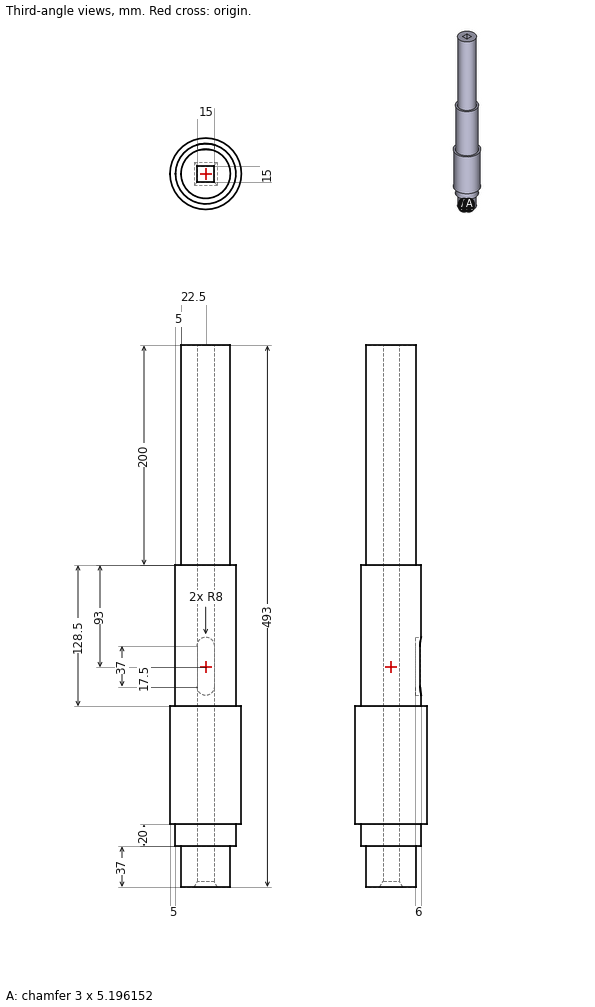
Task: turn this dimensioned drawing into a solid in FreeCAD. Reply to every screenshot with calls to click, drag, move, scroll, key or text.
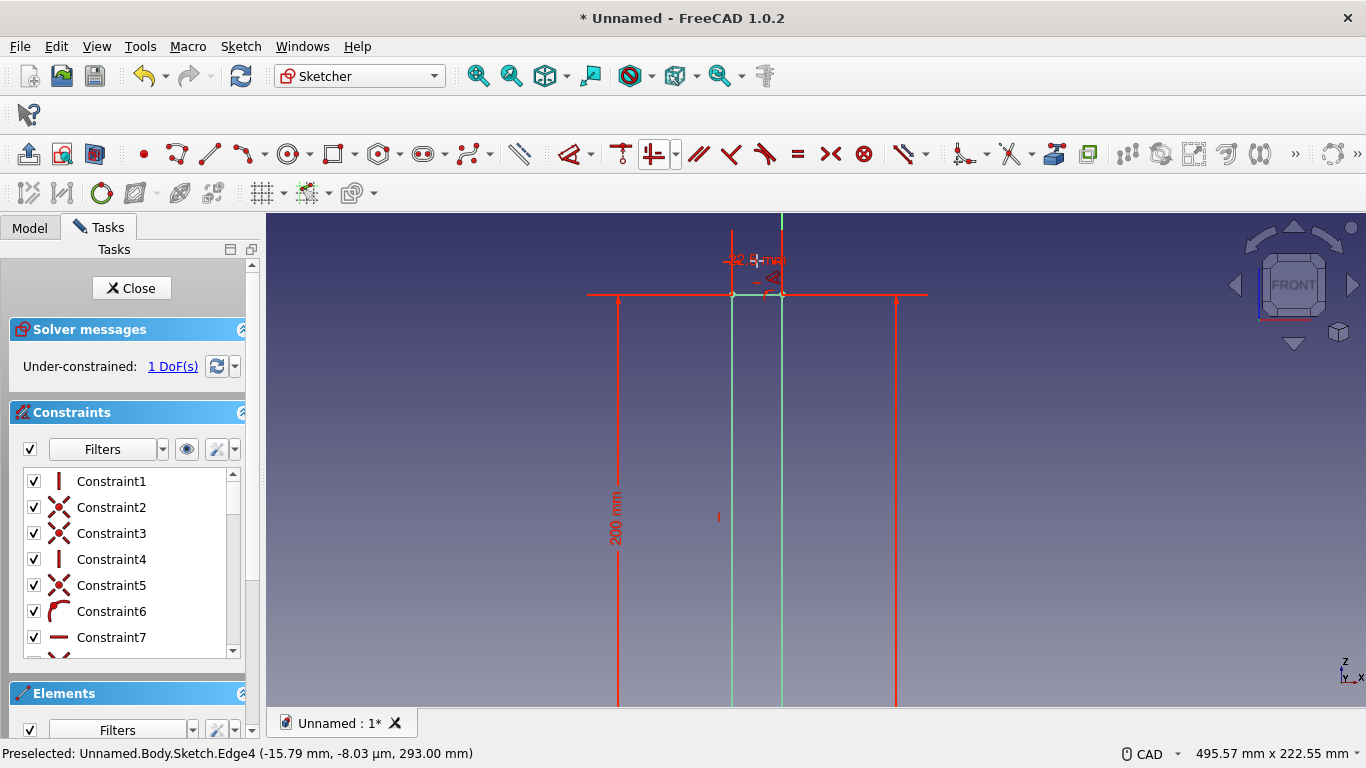
scroll(748, 295, down, 6)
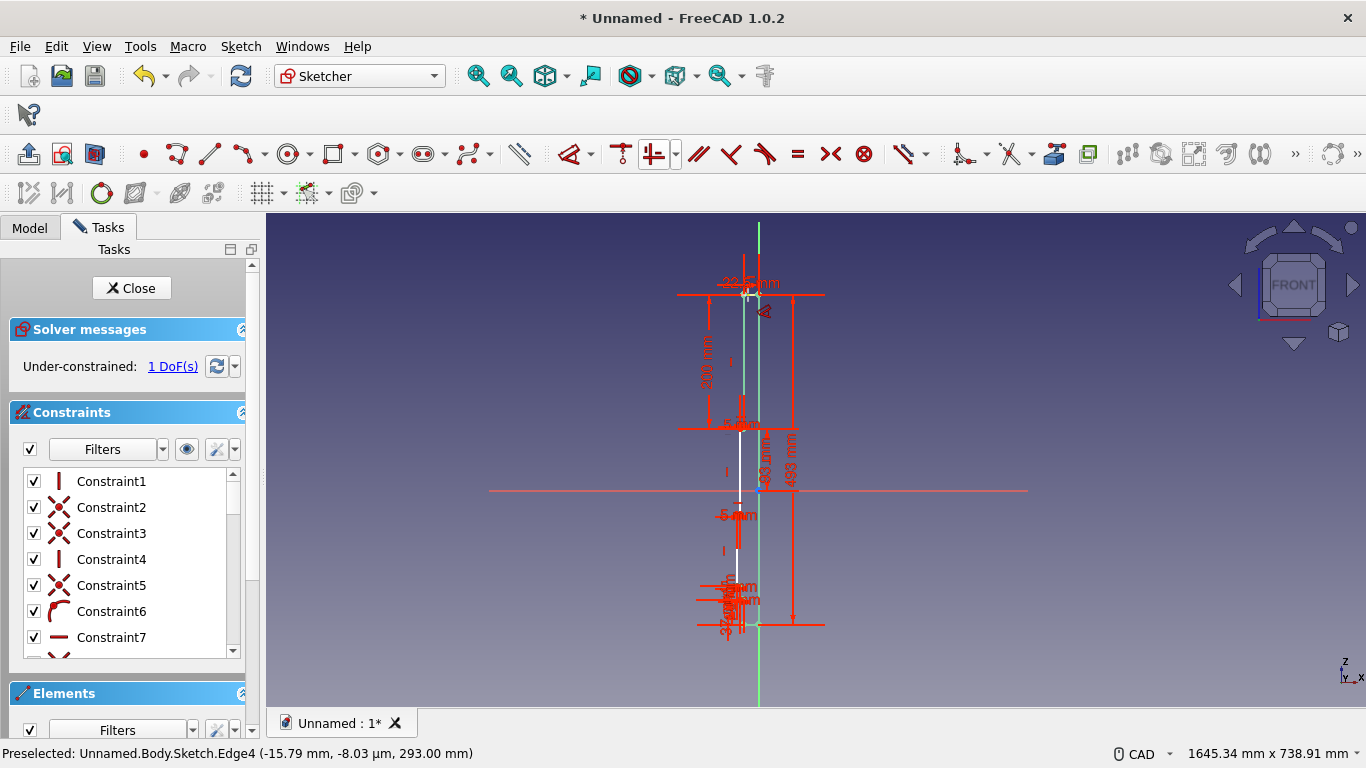
click(740, 454)
click(682, 472)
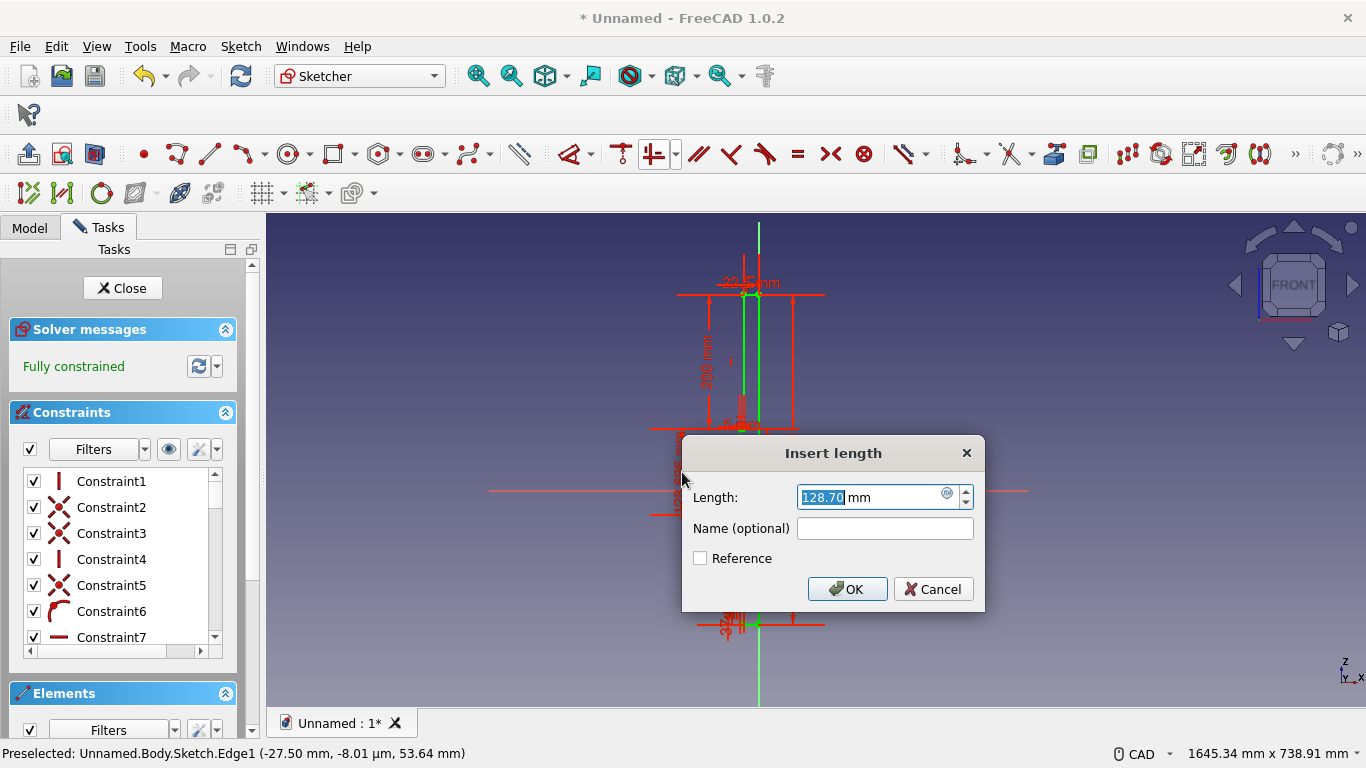
text(128.5)
key(Return)
key(Escape)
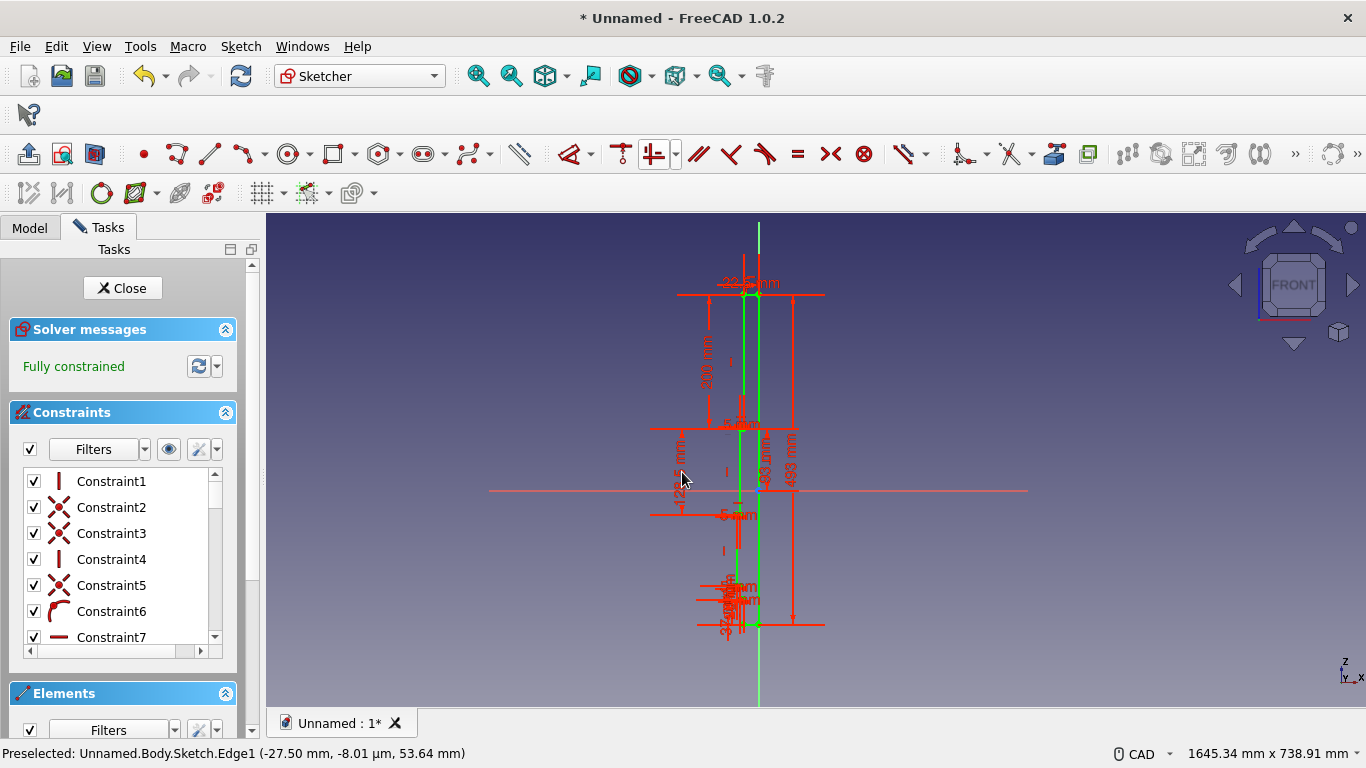
click(123, 288)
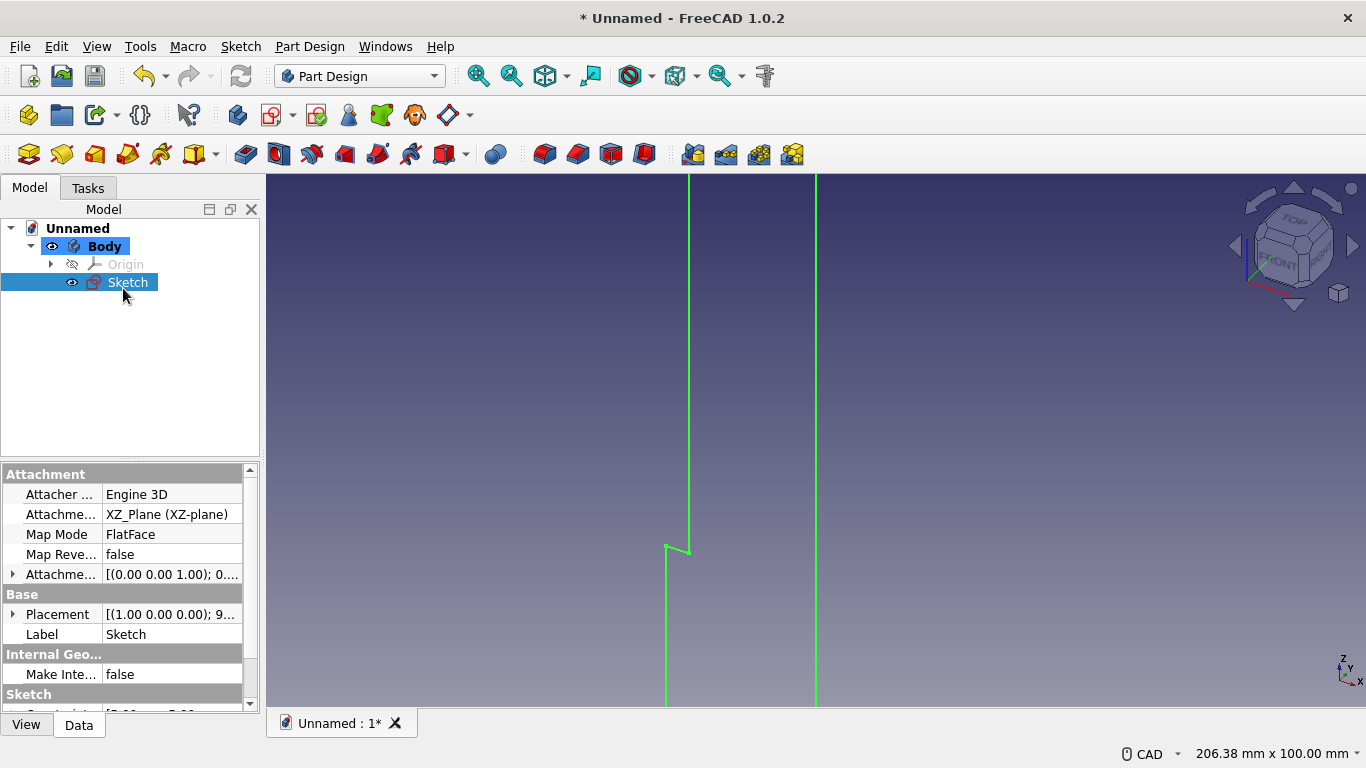
click(62, 154)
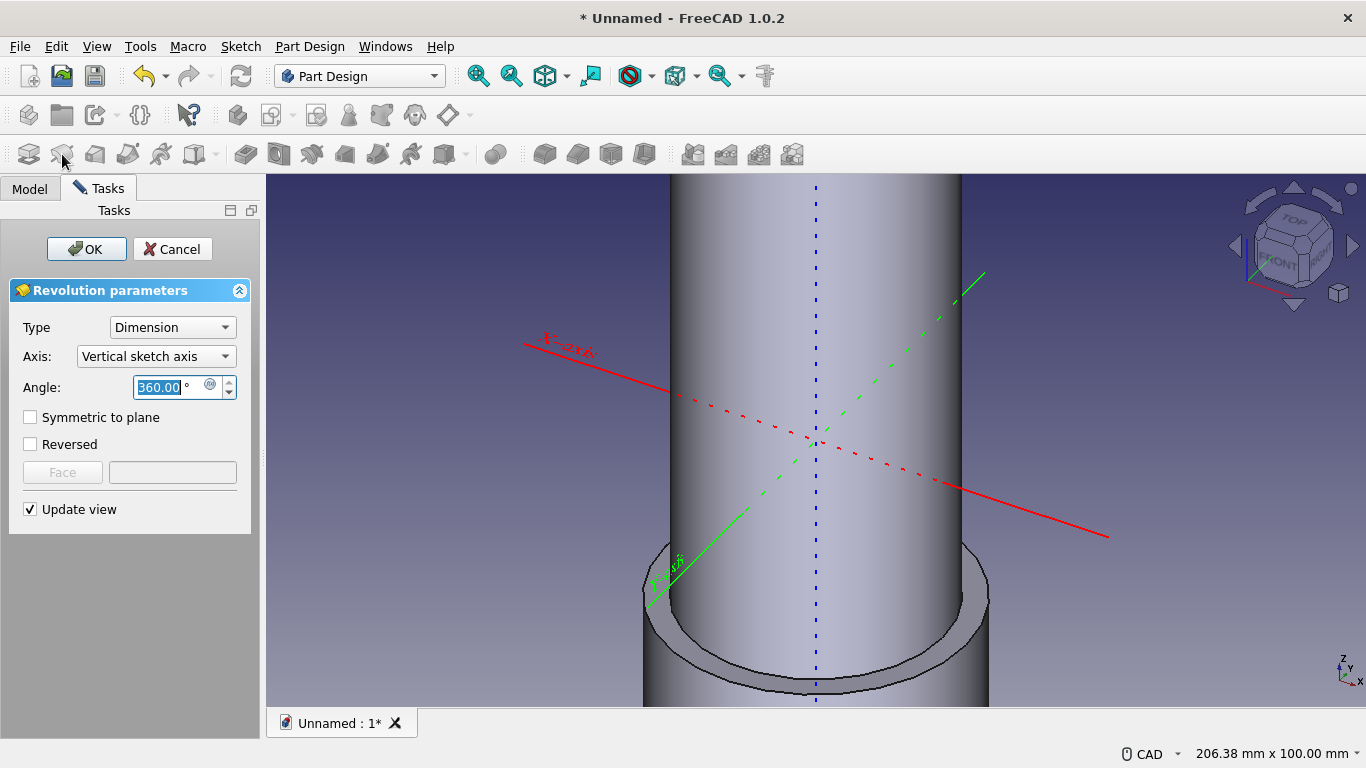
click(87, 249)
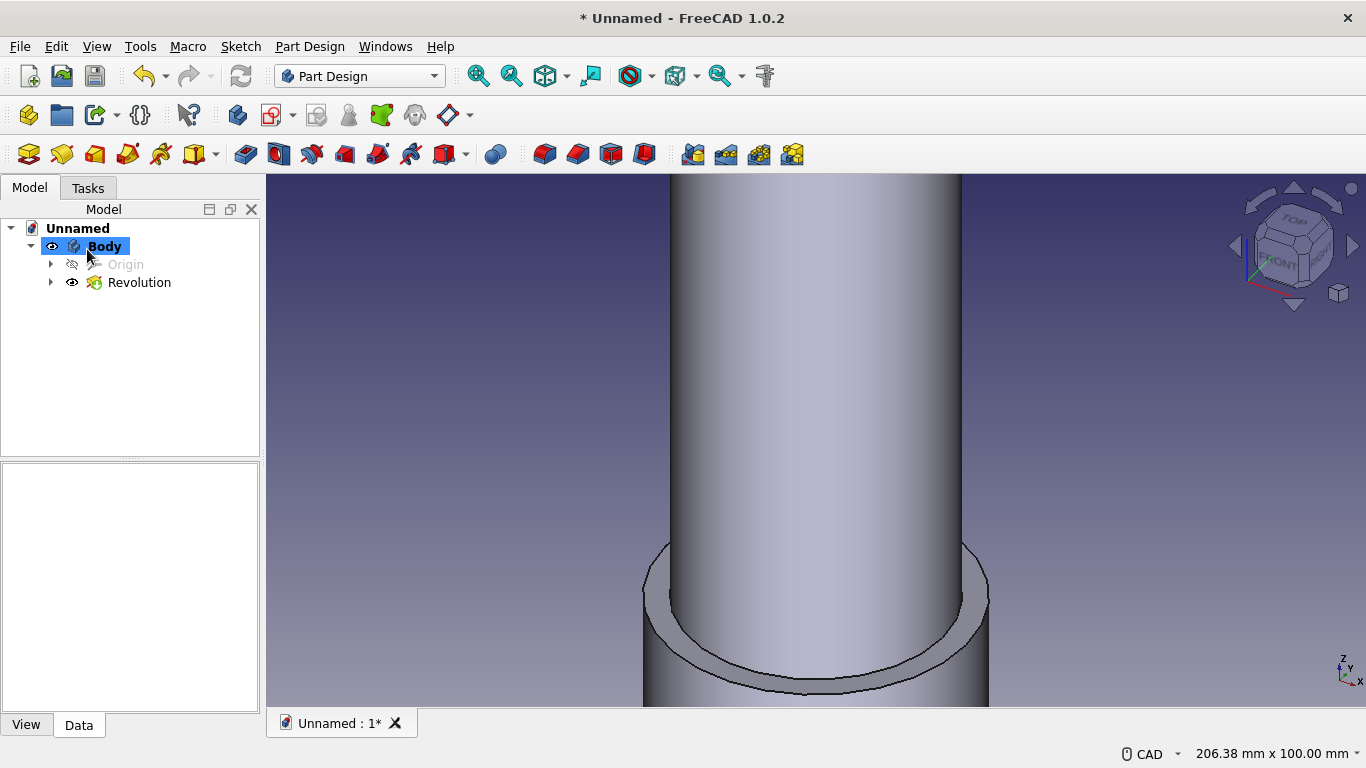
click(479, 76)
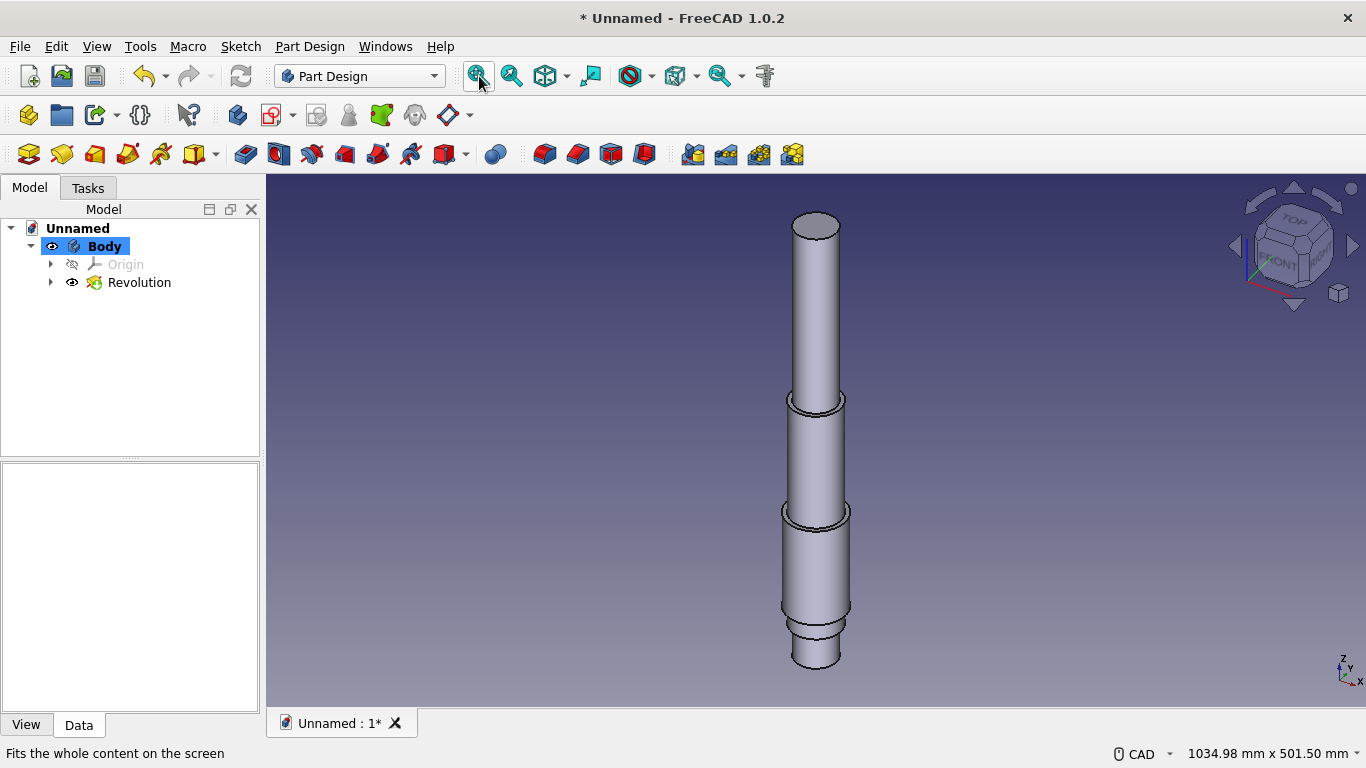
key(5)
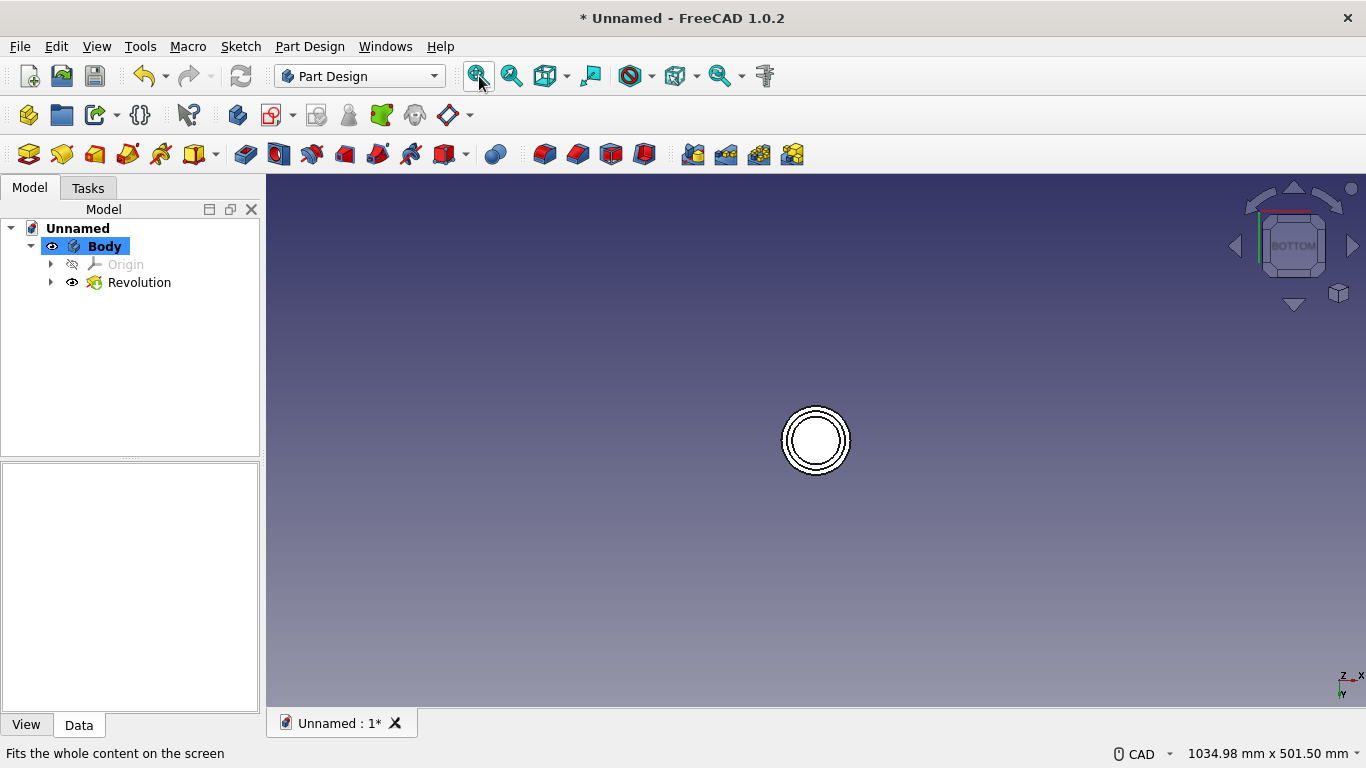
click(479, 76)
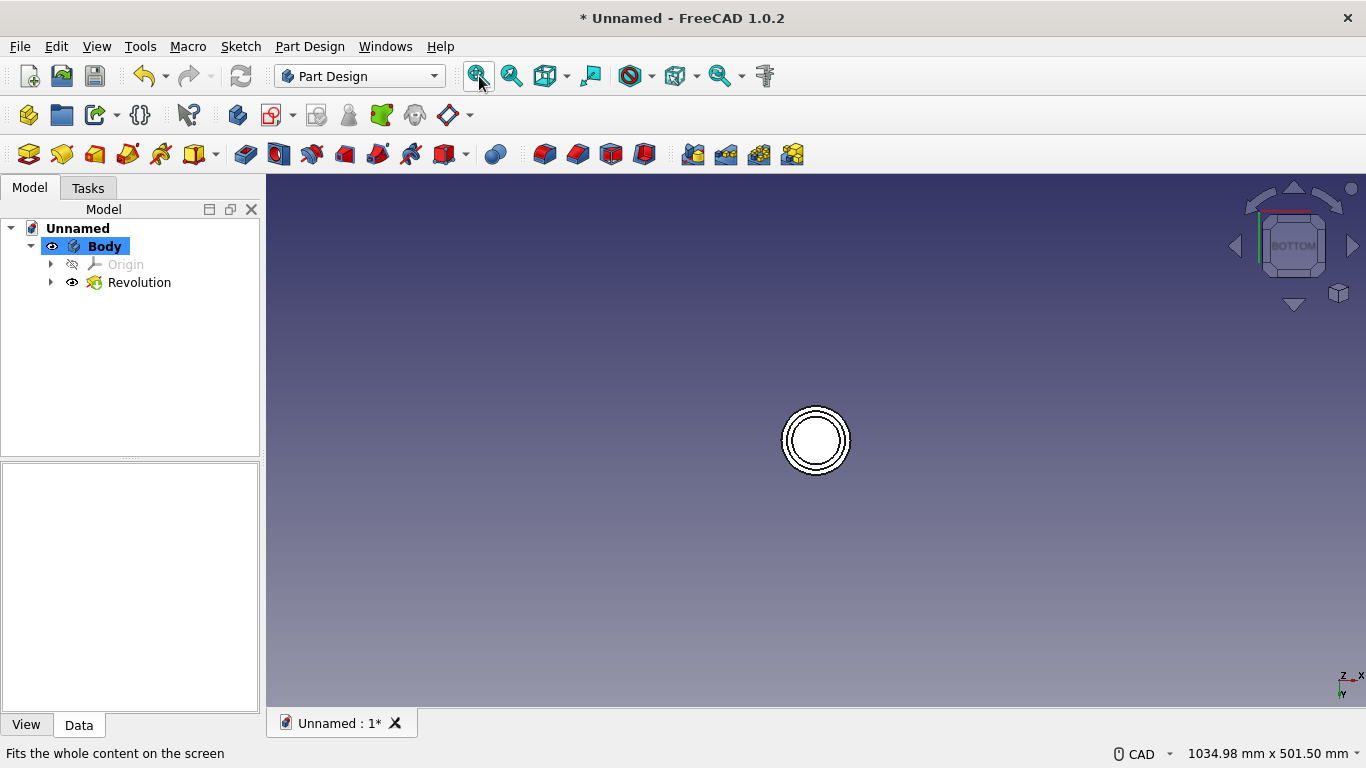
click(816, 439)